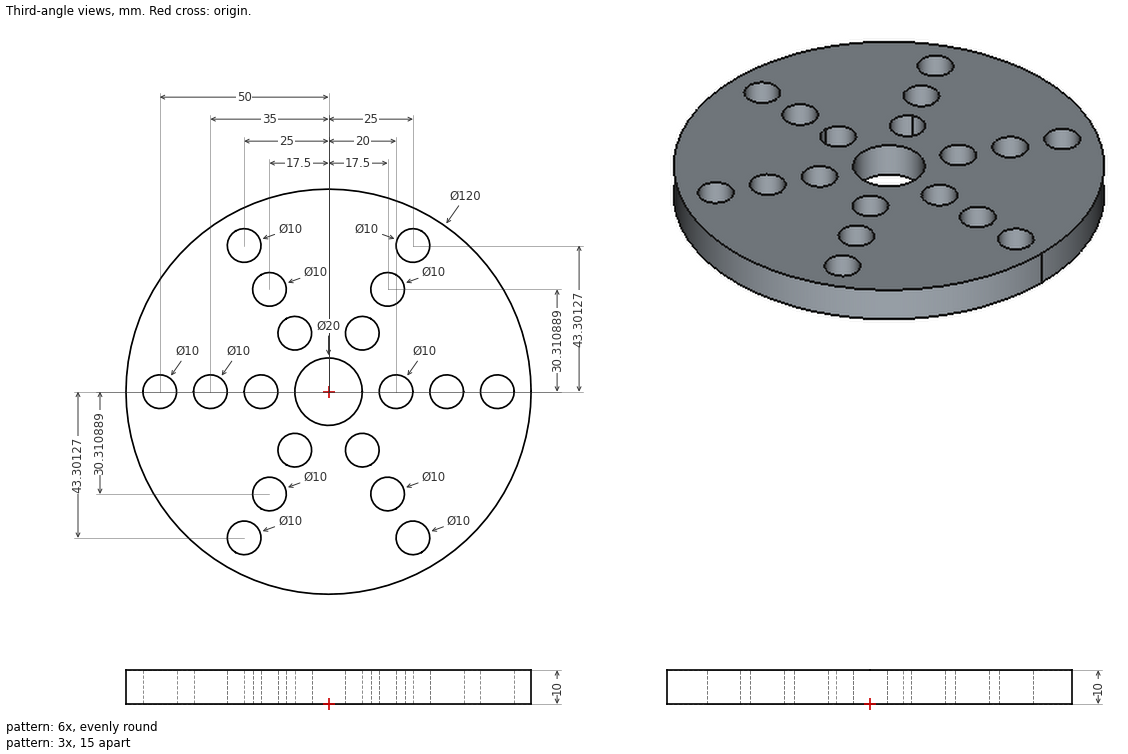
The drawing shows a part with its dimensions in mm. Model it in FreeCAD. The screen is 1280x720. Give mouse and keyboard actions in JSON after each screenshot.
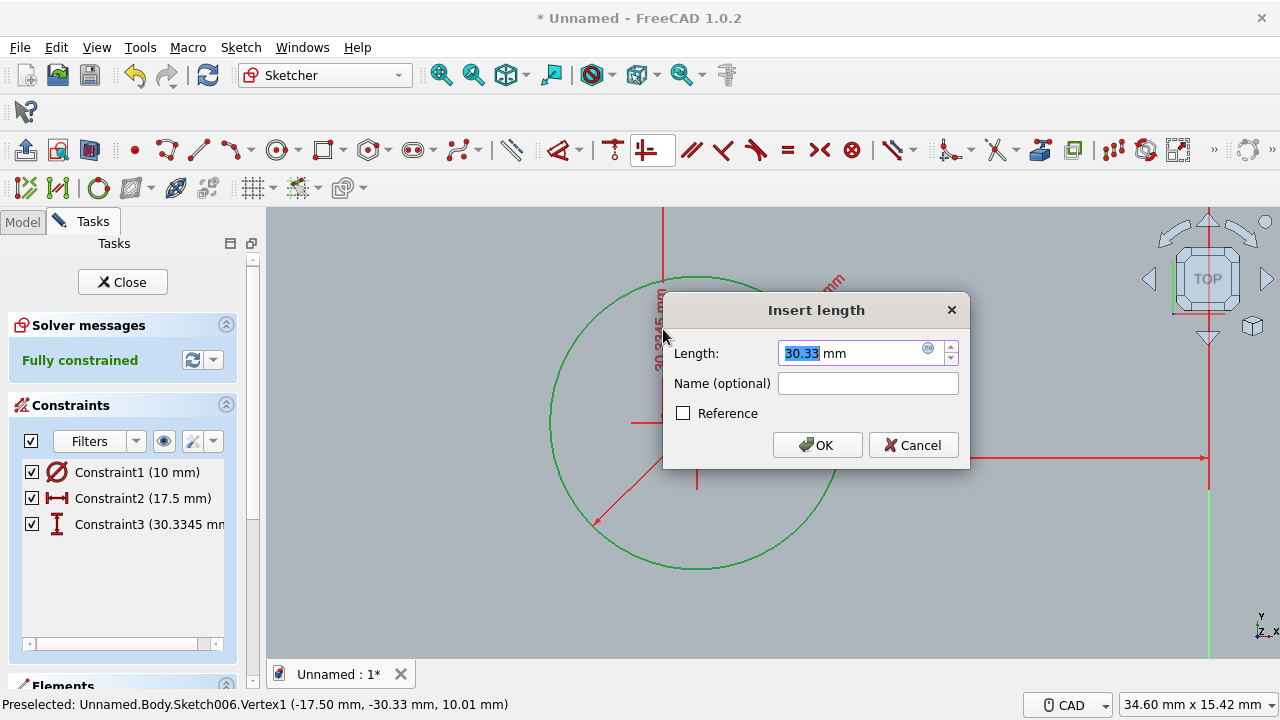
{"action": "type", "text": "30.310889"}
{"action": "key", "text": "Return"}
{"action": "key", "text": "Escape"}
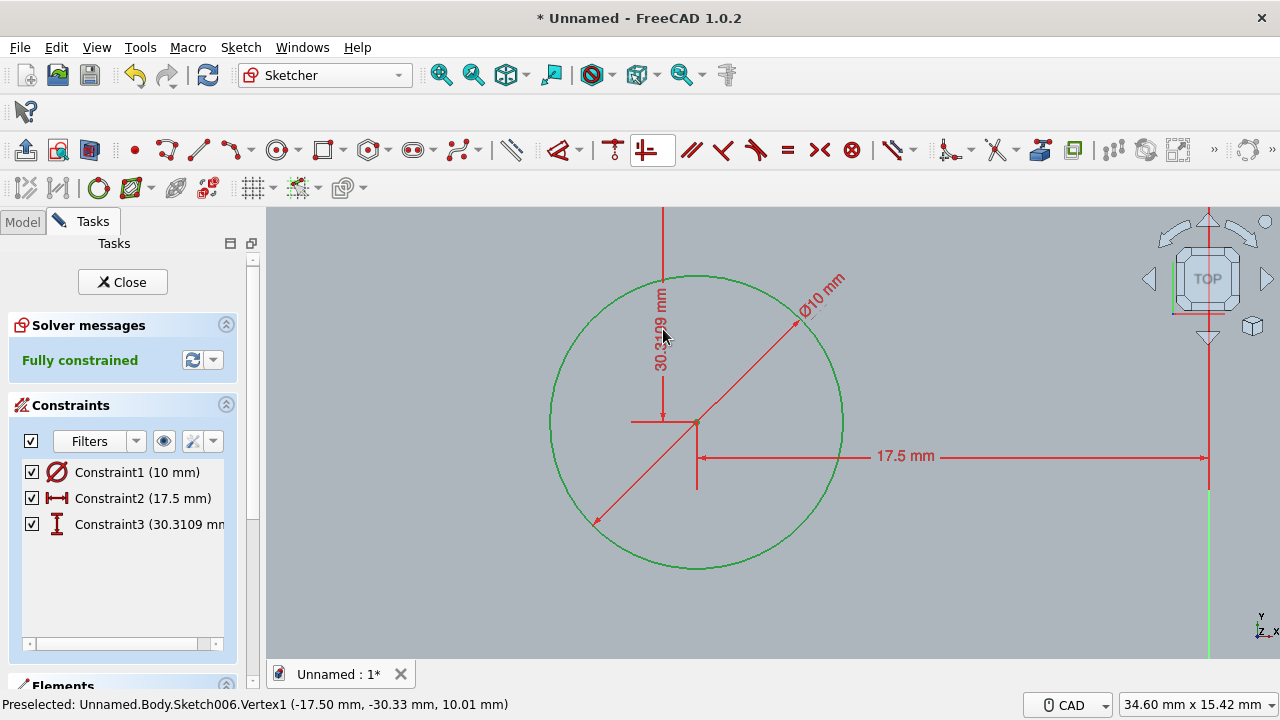
{"action": "left_click", "coordinate": [123, 282]}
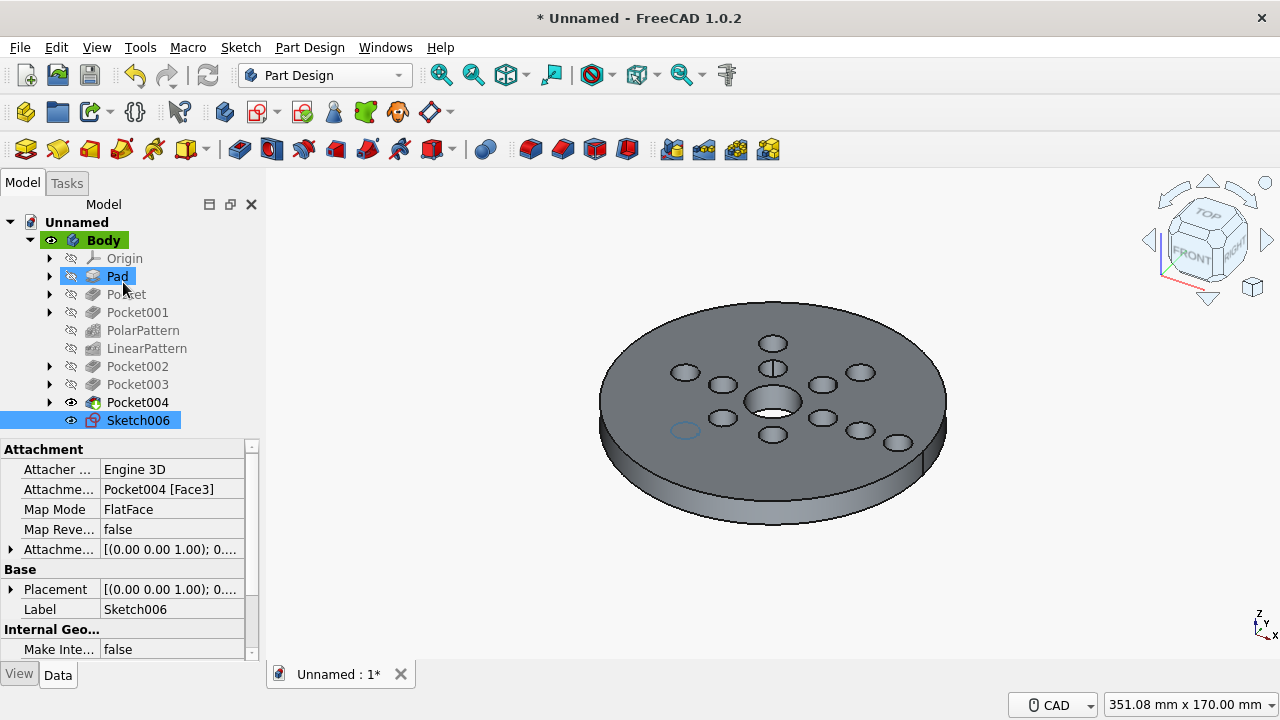
{"action": "left_click", "coordinate": [240, 150]}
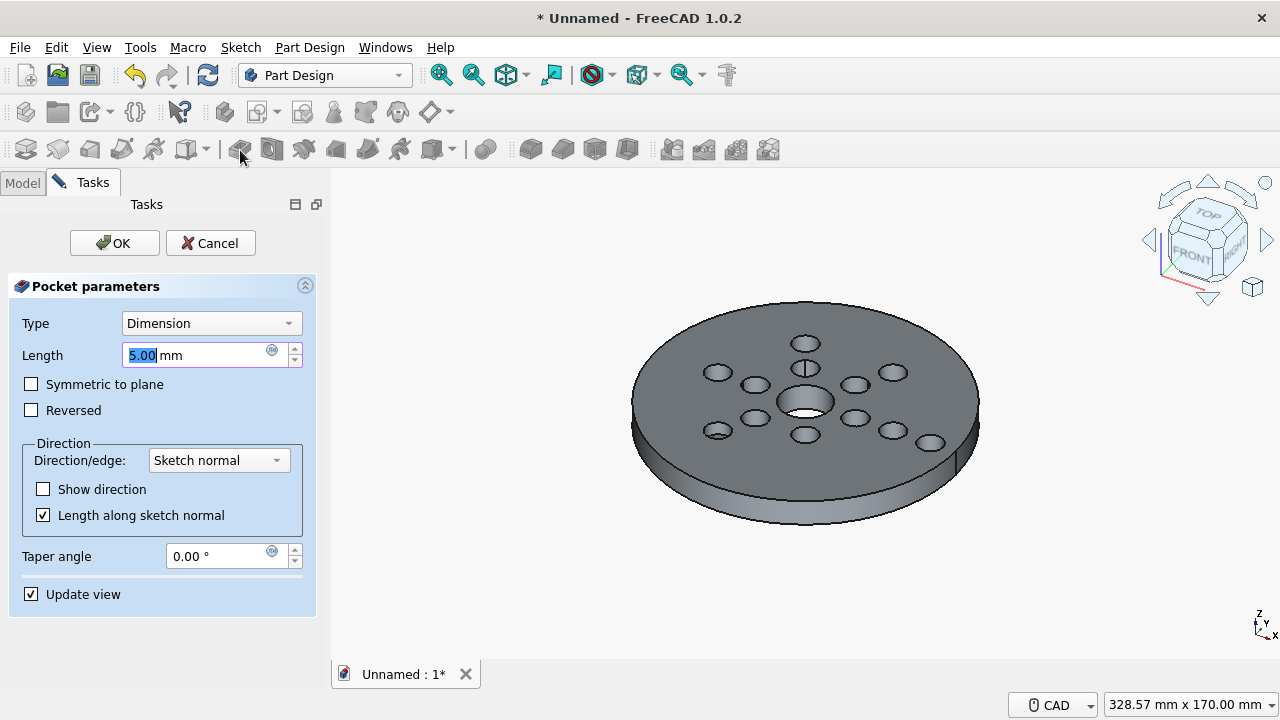
{"action": "type", "text": "10"}
{"action": "key", "text": "Tab"}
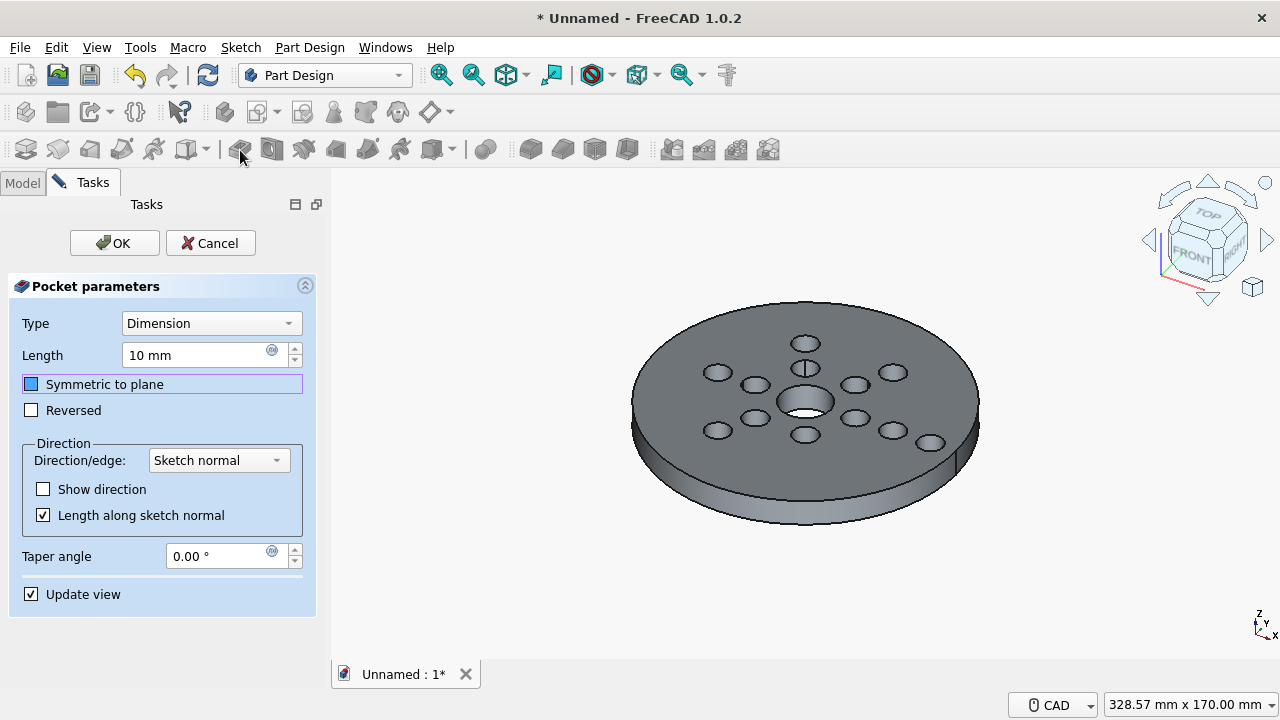
{"action": "left_click", "coordinate": [115, 243]}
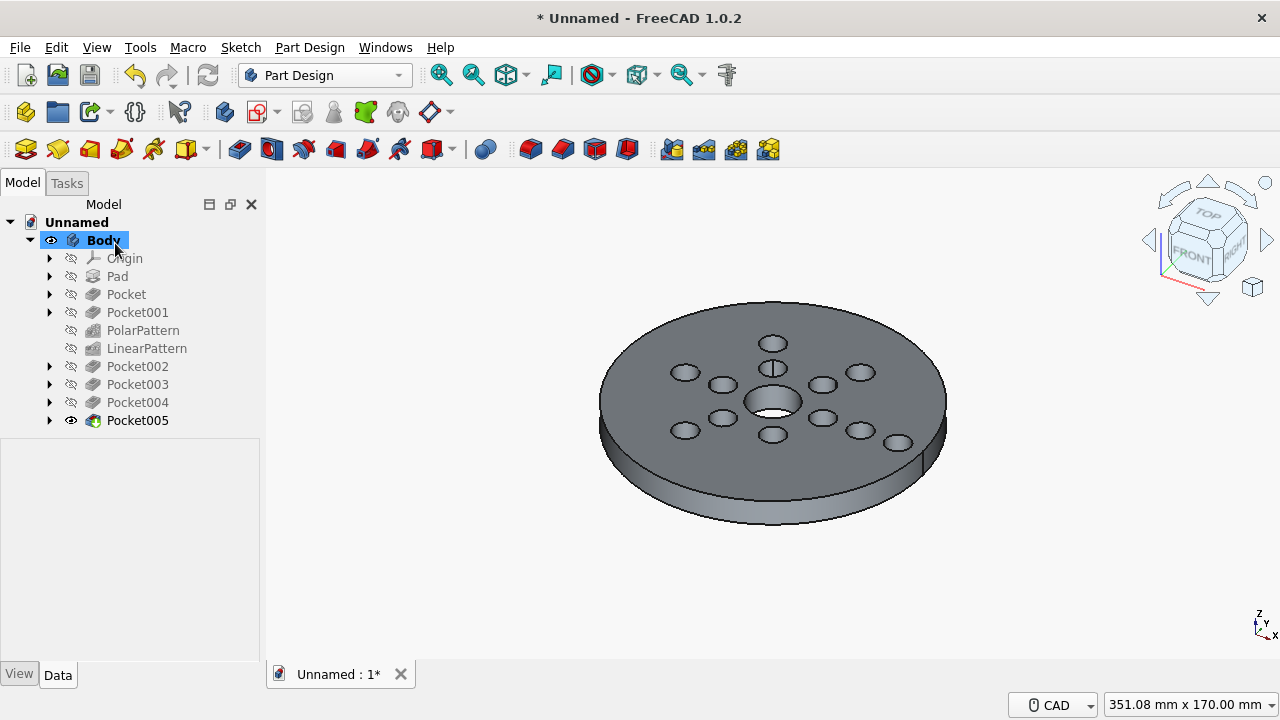
{"action": "left_click", "coordinate": [766, 464]}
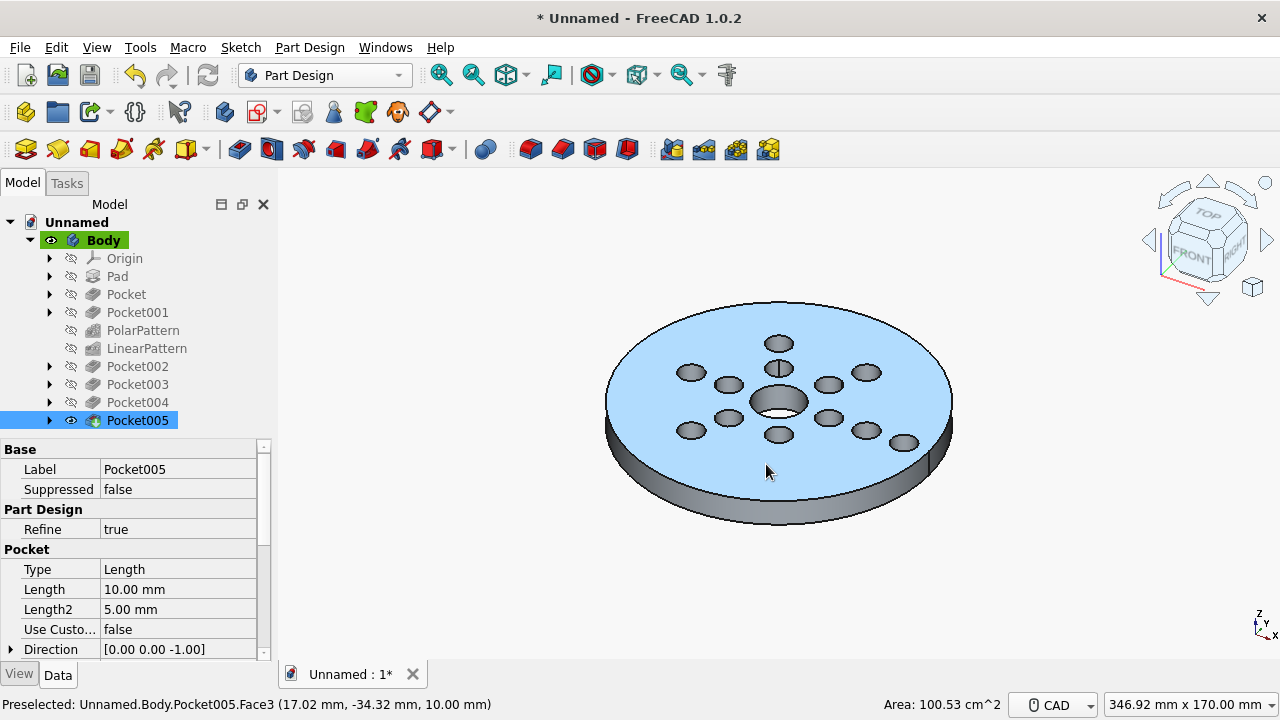
{"action": "left_click", "coordinate": [258, 112]}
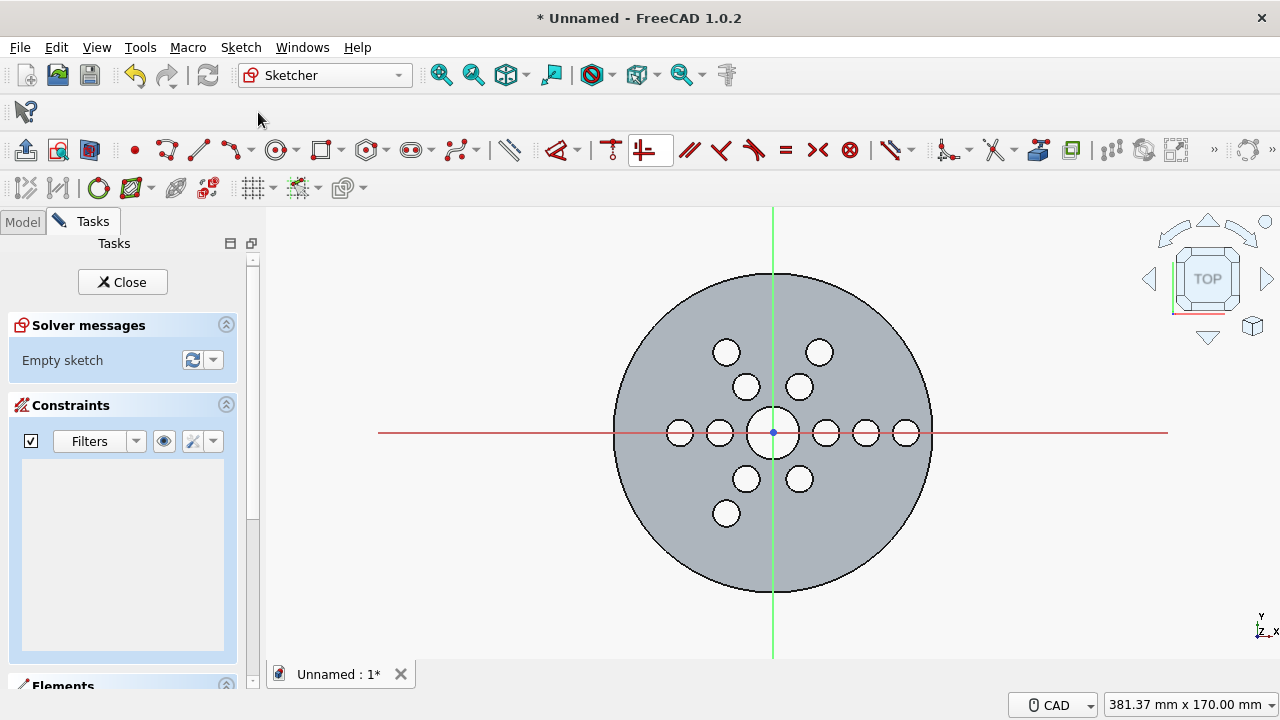
{"action": "scroll", "coordinate": [831, 522], "scroll_direction": "up", "scroll_amount": 12}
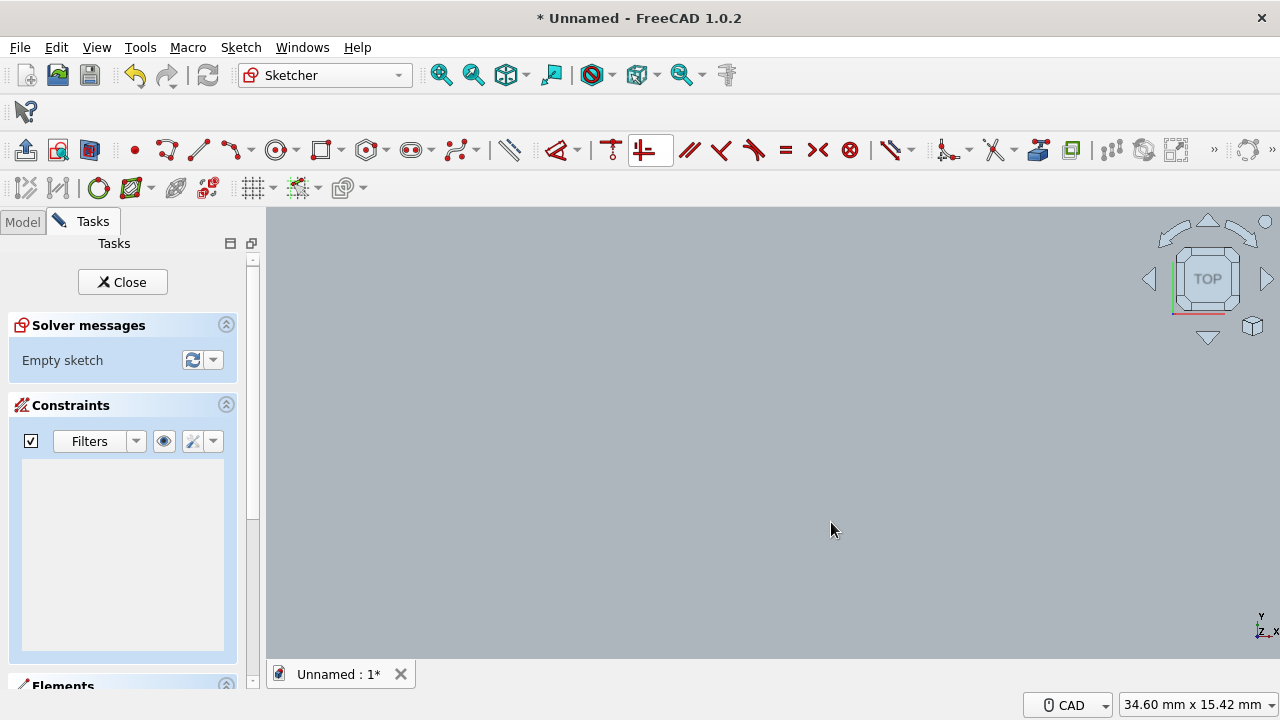
{"action": "left_click", "coordinate": [276, 150]}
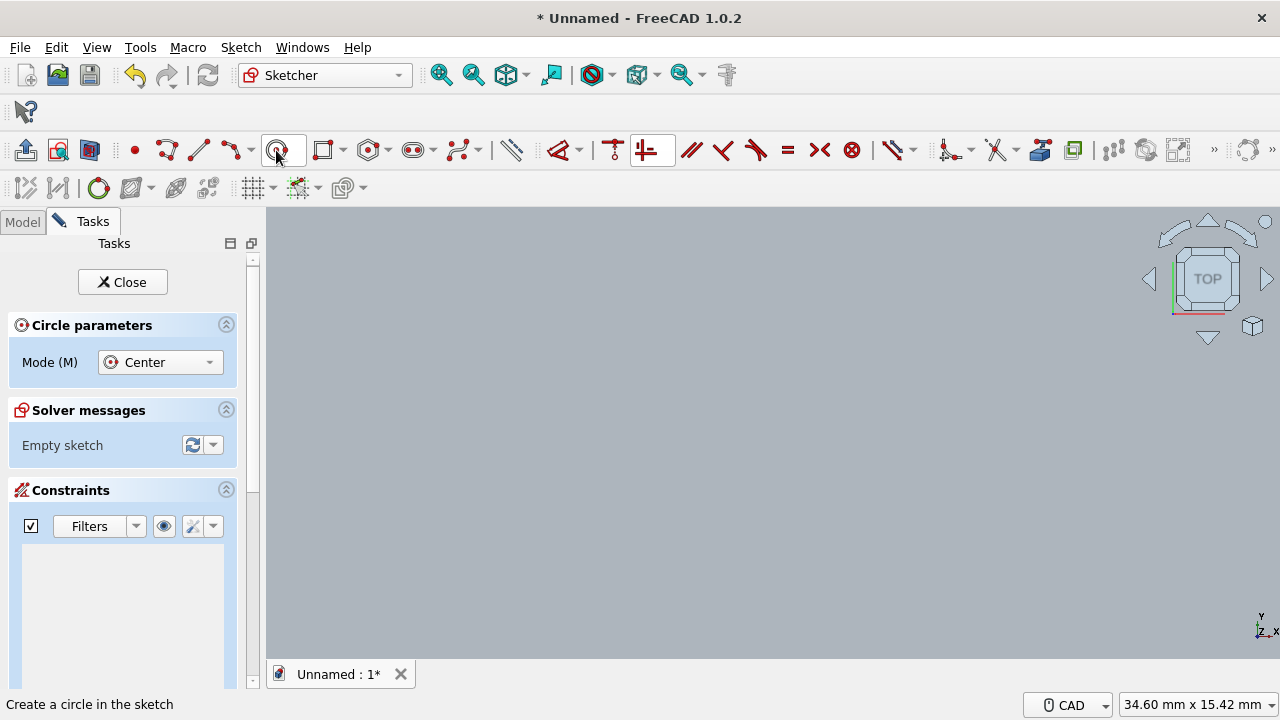
{"action": "left_click", "coordinate": [699, 422]}
{"action": "left_click", "coordinate": [803, 319]}
{"action": "key", "text": "Escape"}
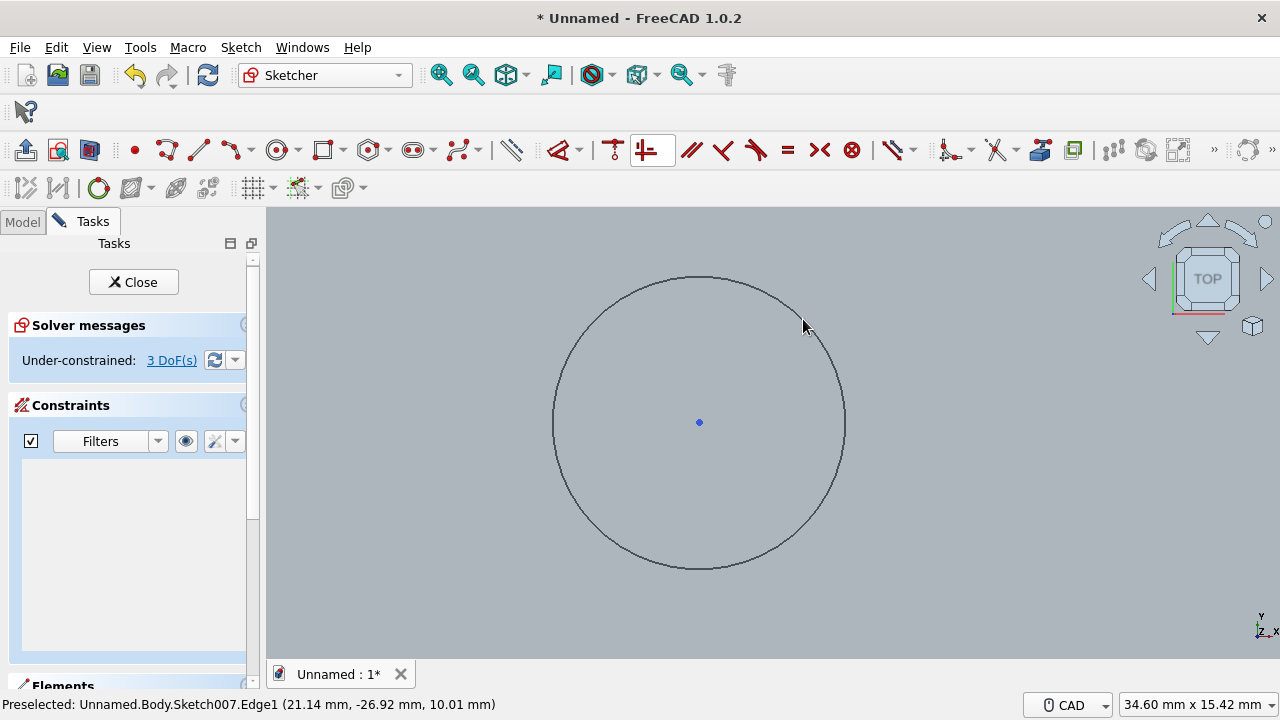
{"action": "key", "text": "d"}